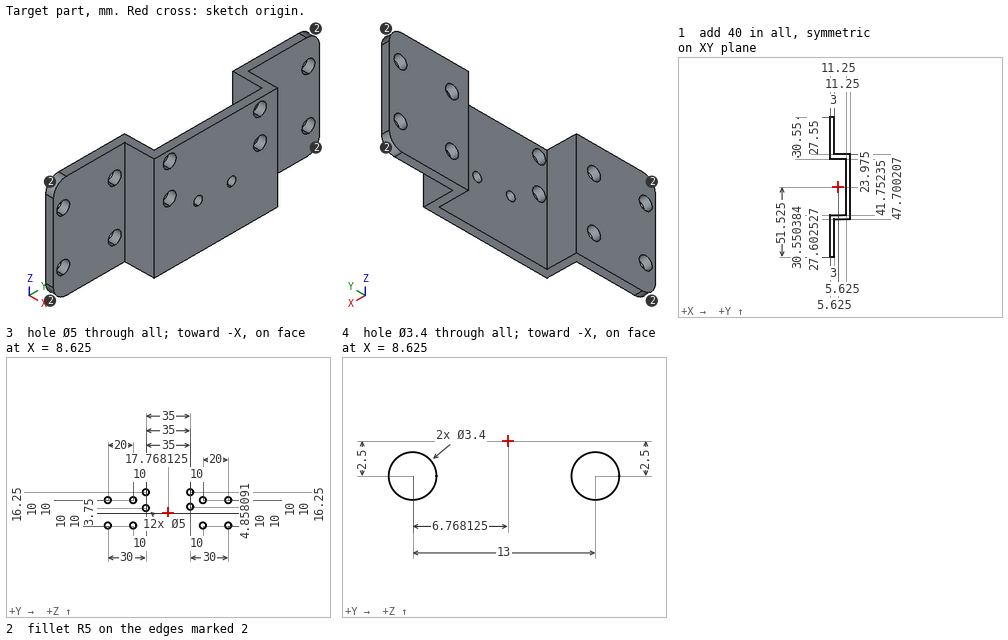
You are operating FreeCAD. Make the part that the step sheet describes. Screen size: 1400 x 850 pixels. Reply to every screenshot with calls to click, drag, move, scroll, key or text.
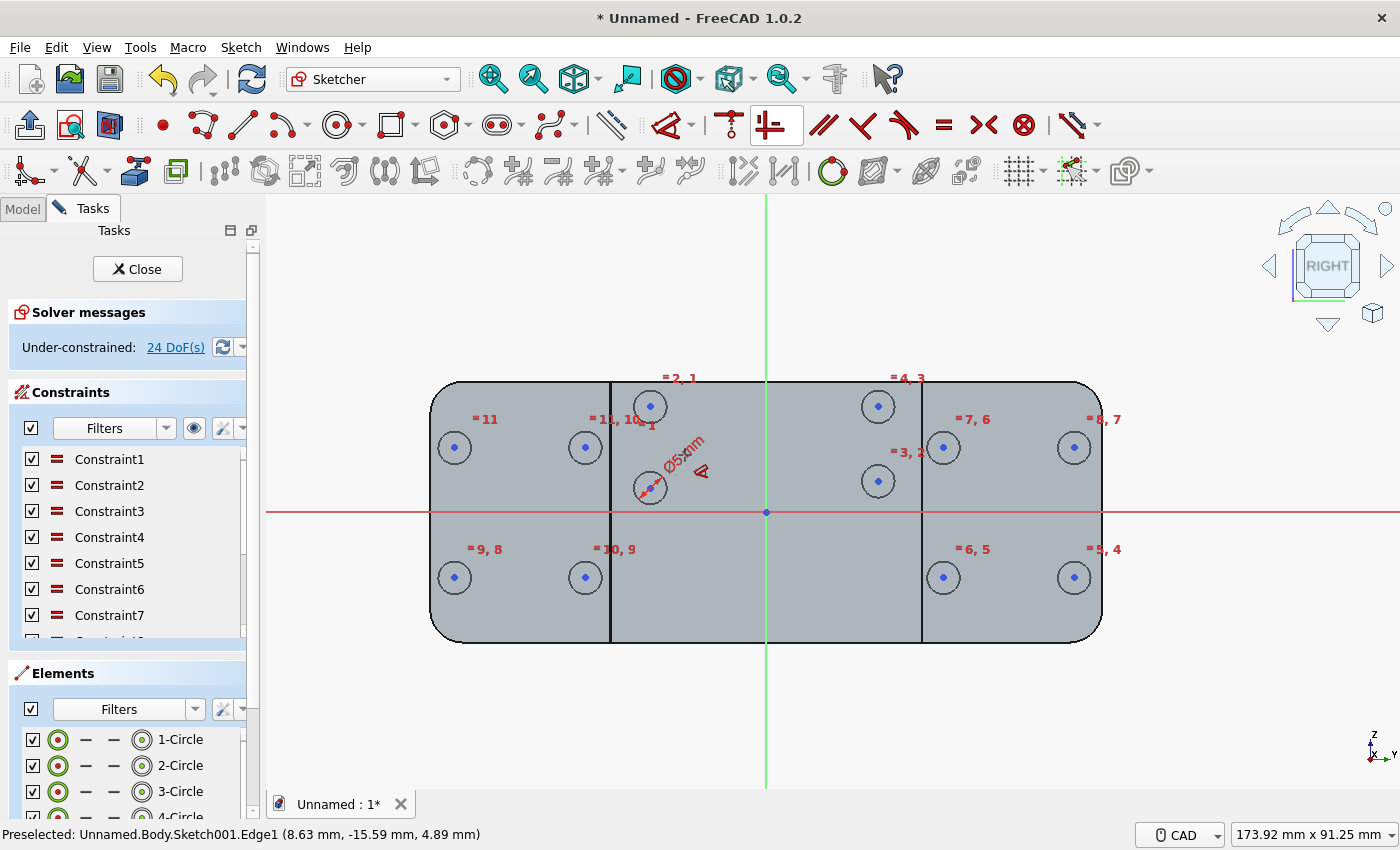
click(1074, 578)
click(1108, 545)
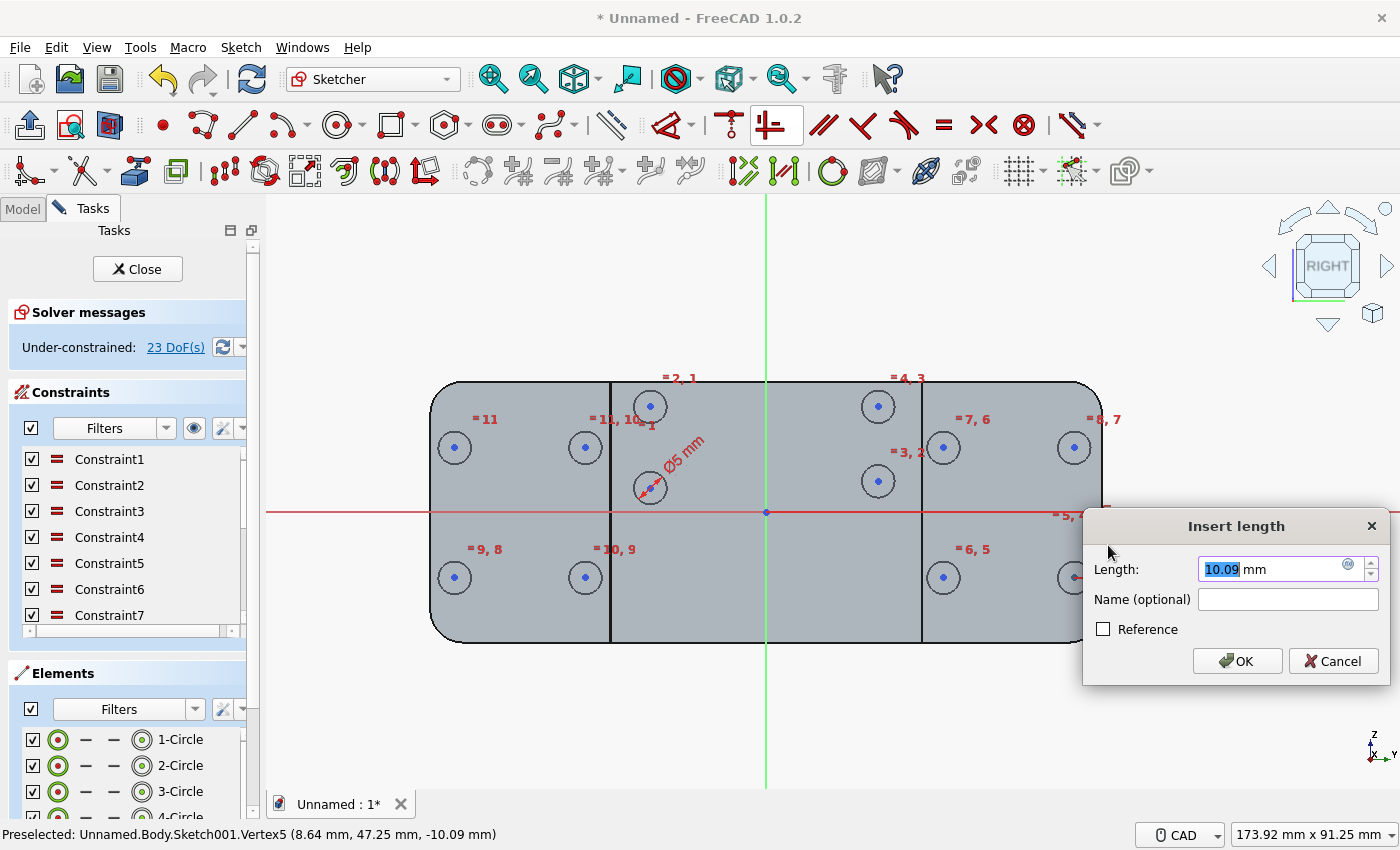
text(10)
key(Return)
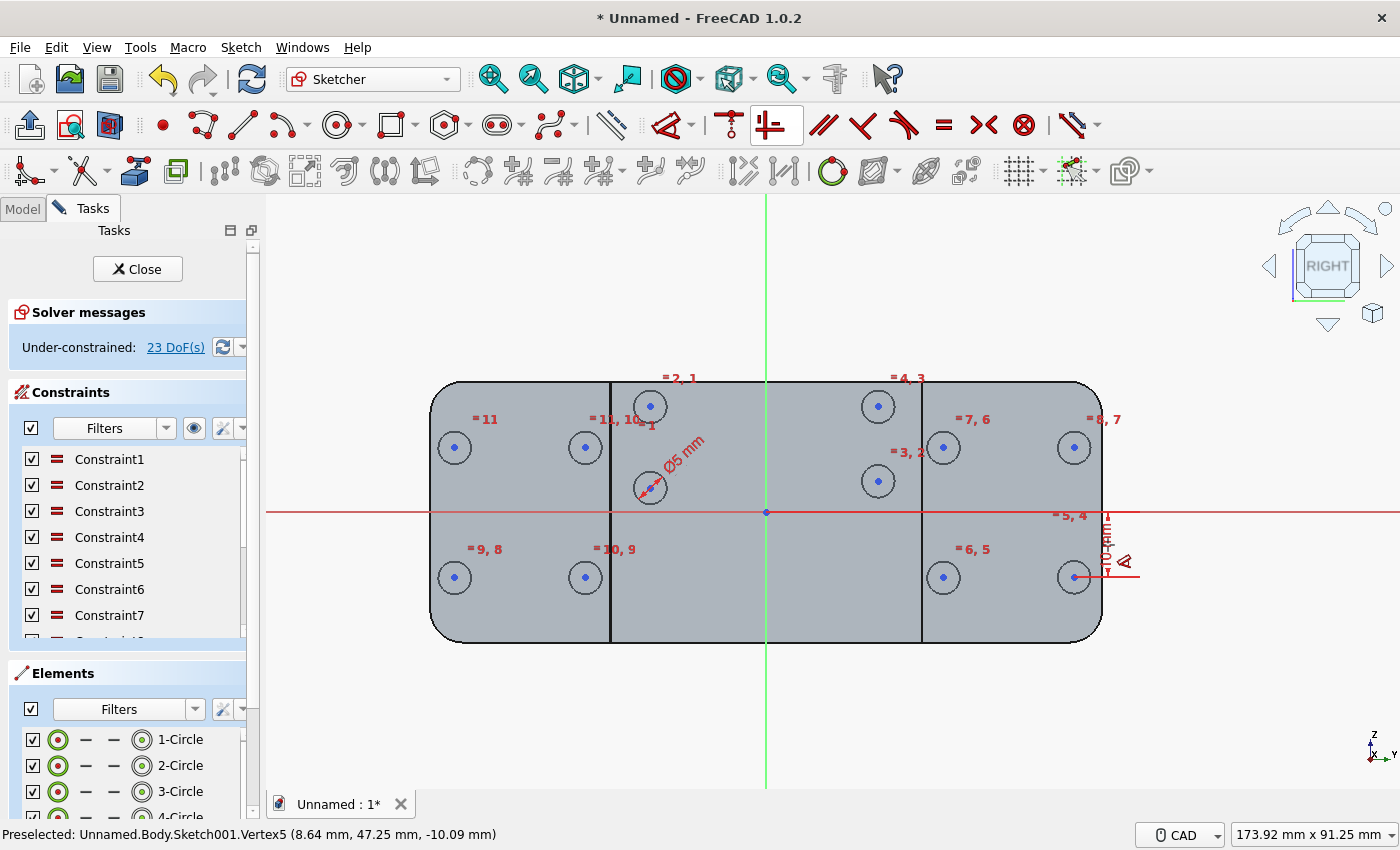
click(944, 578)
click(978, 545)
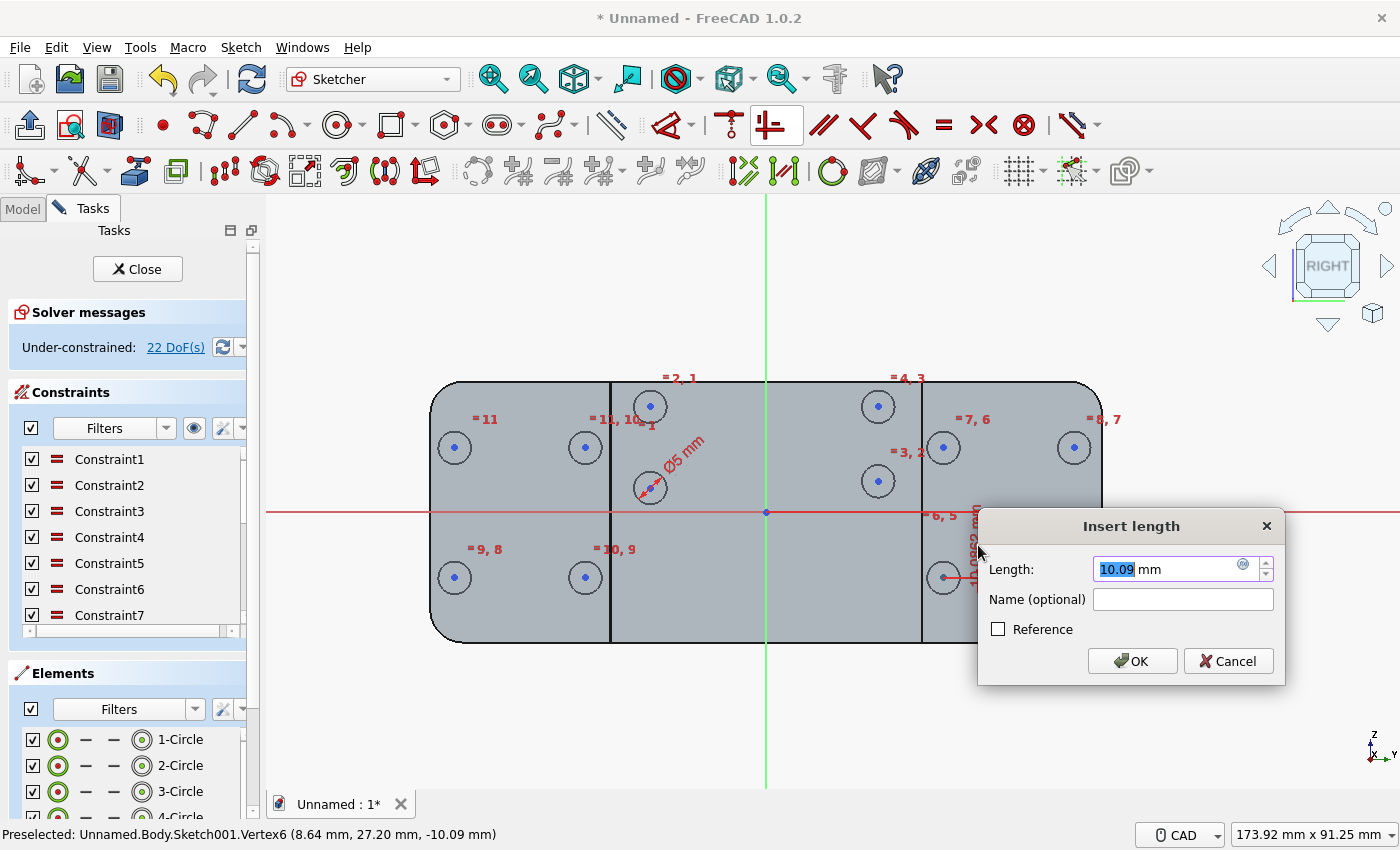
text(10)
key(Return)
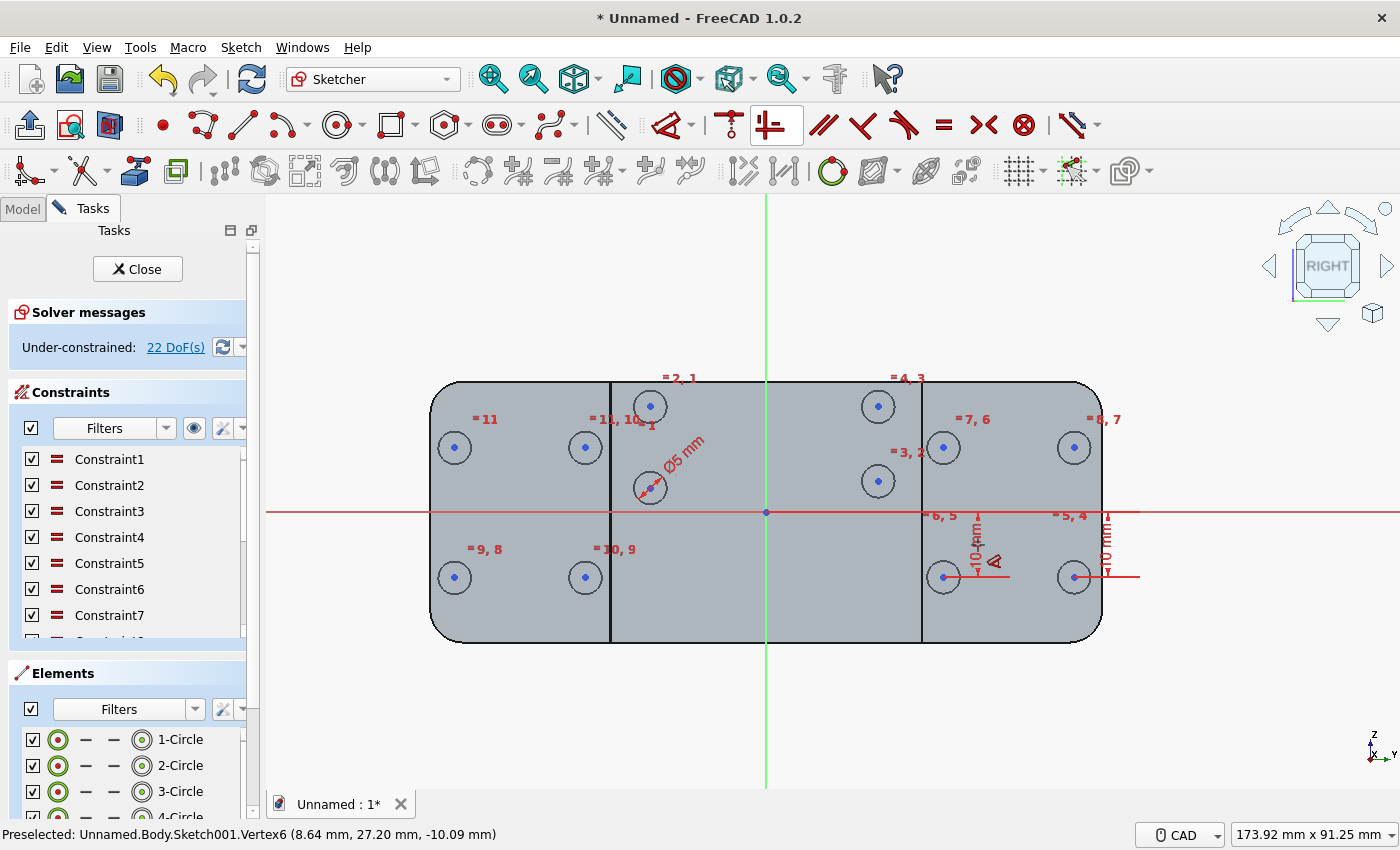
click(944, 448)
click(978, 480)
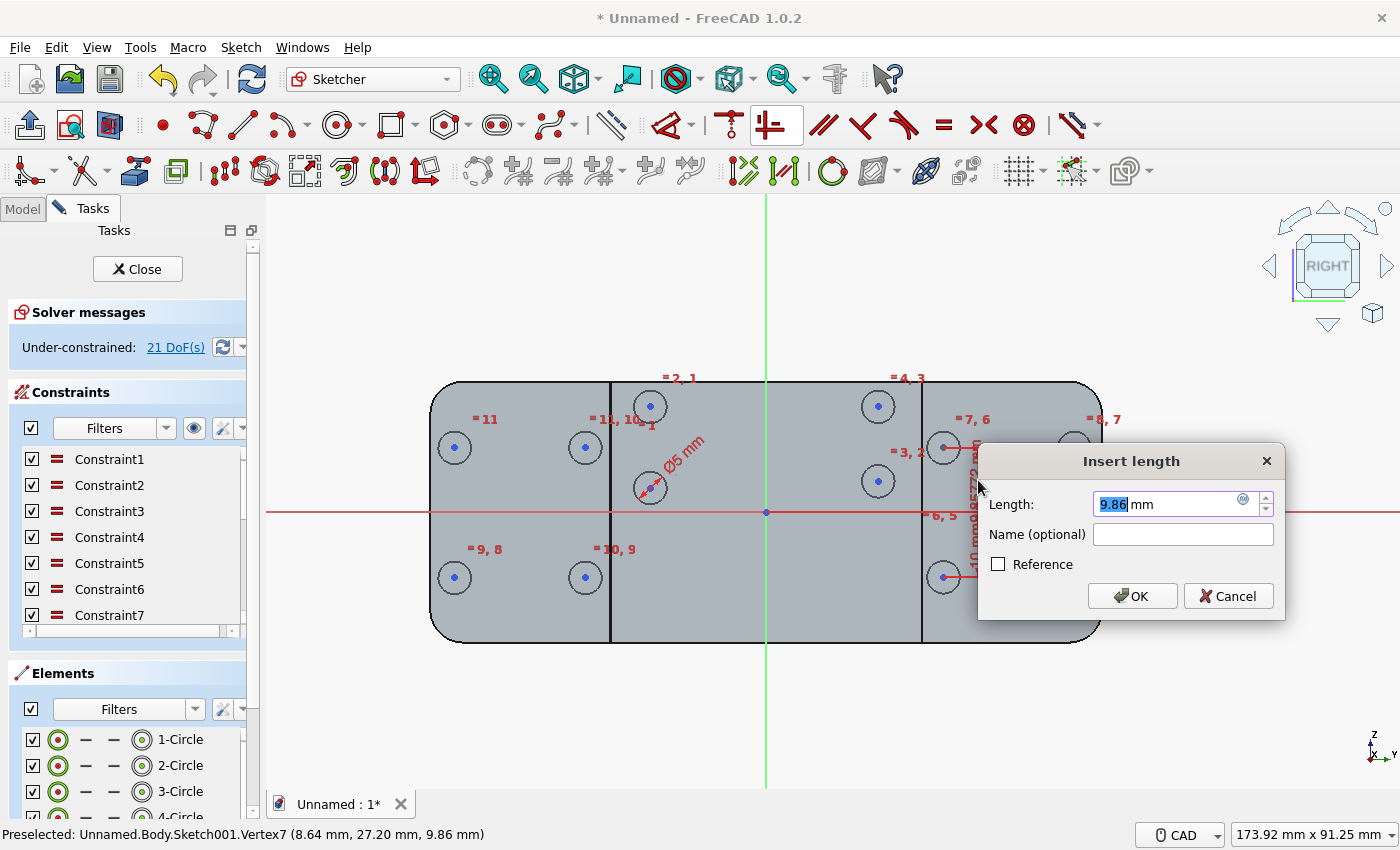
text(10)
key(Return)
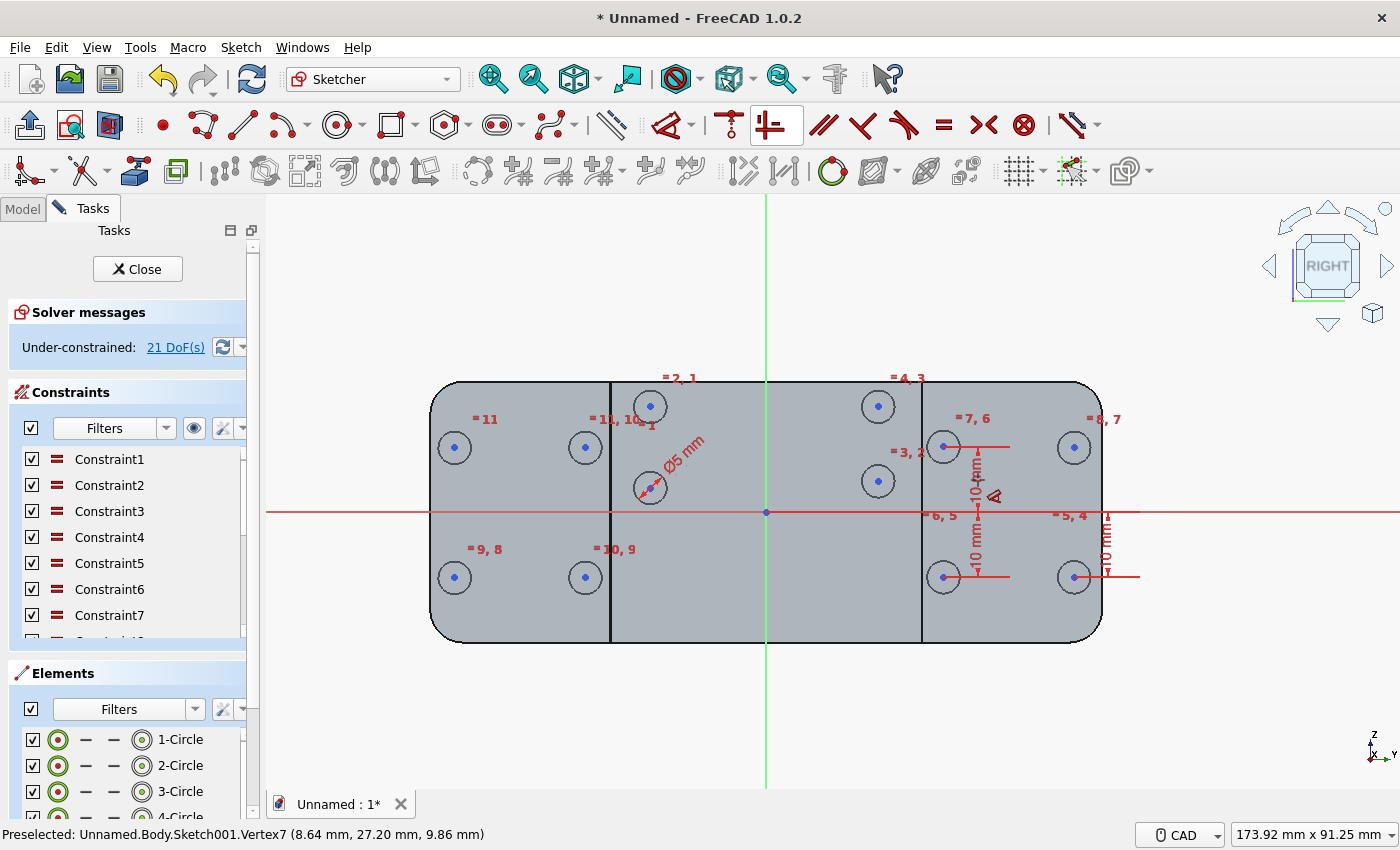
click(1074, 448)
click(1108, 480)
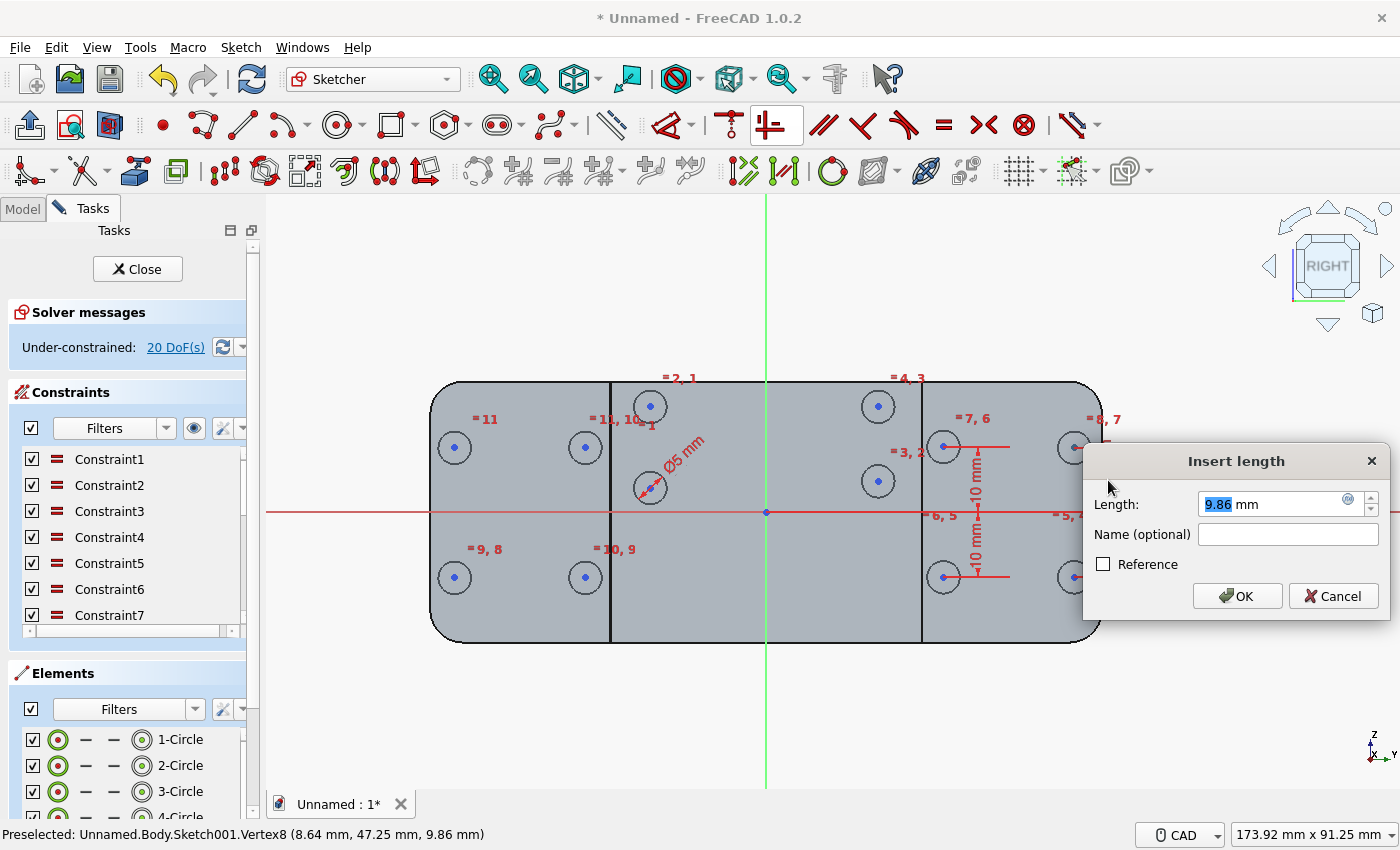
text(10)
key(Return)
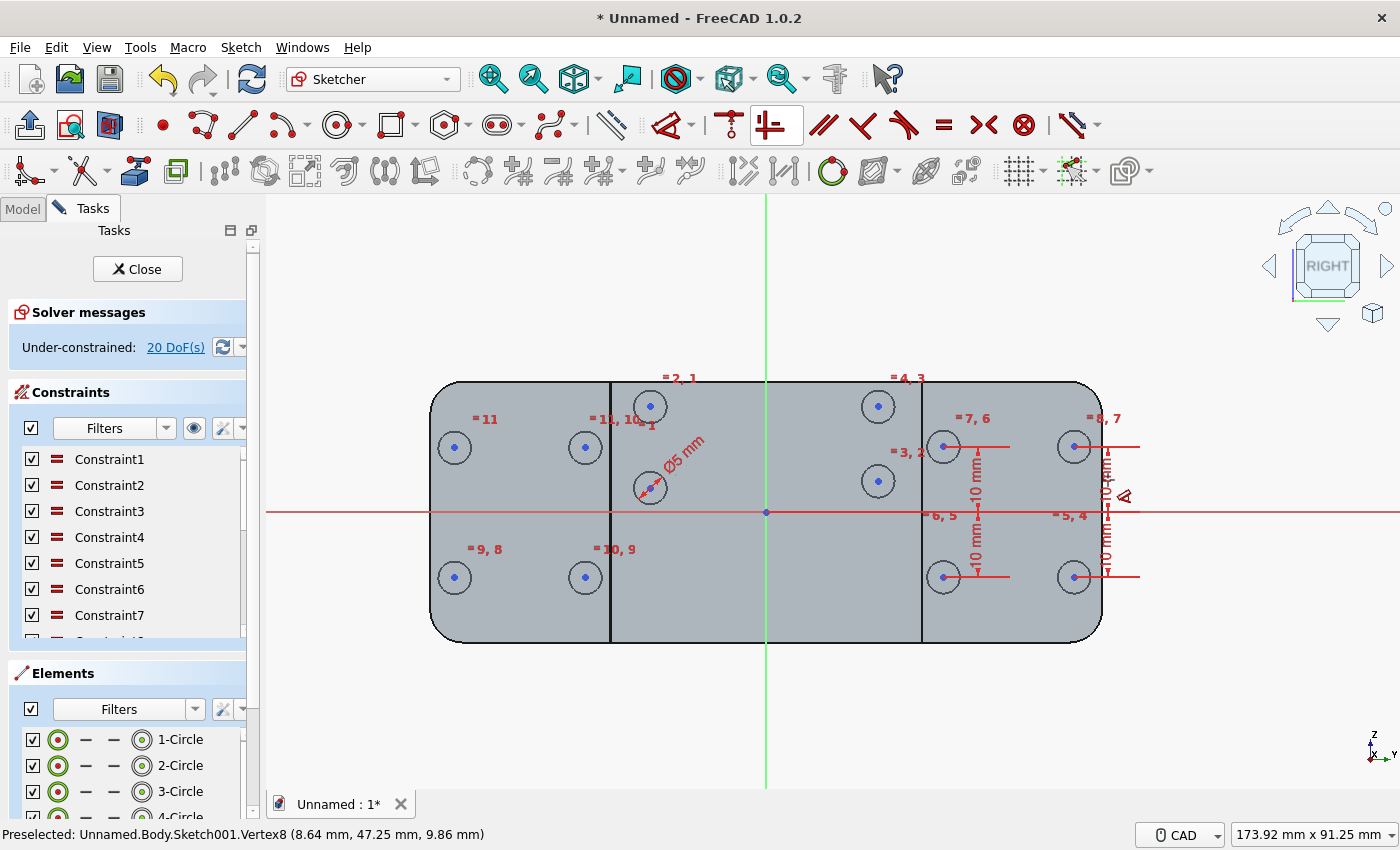
click(455, 578)
click(421, 545)